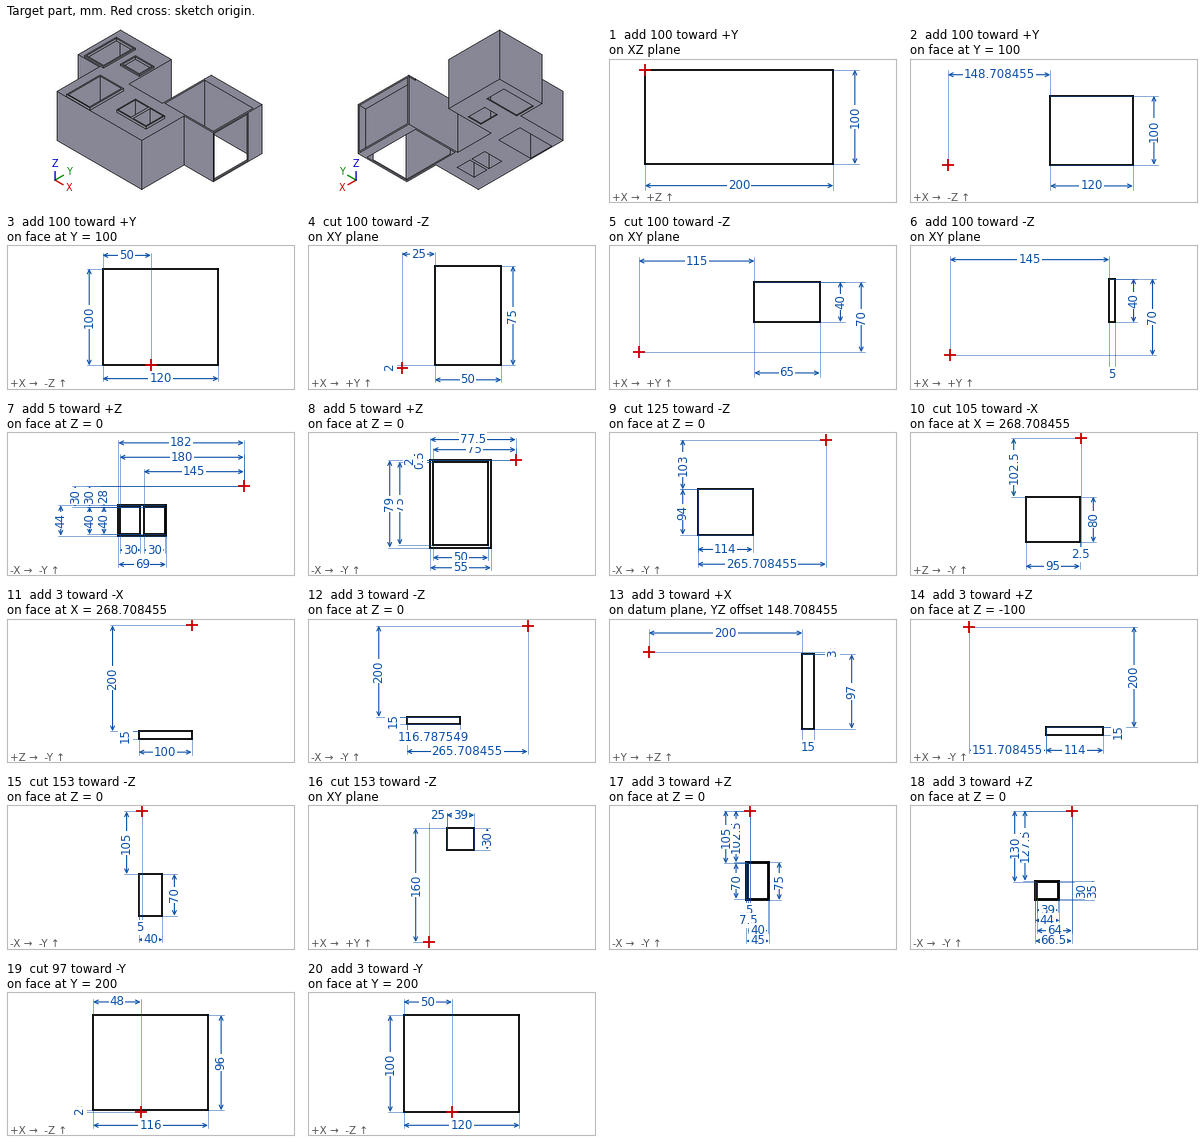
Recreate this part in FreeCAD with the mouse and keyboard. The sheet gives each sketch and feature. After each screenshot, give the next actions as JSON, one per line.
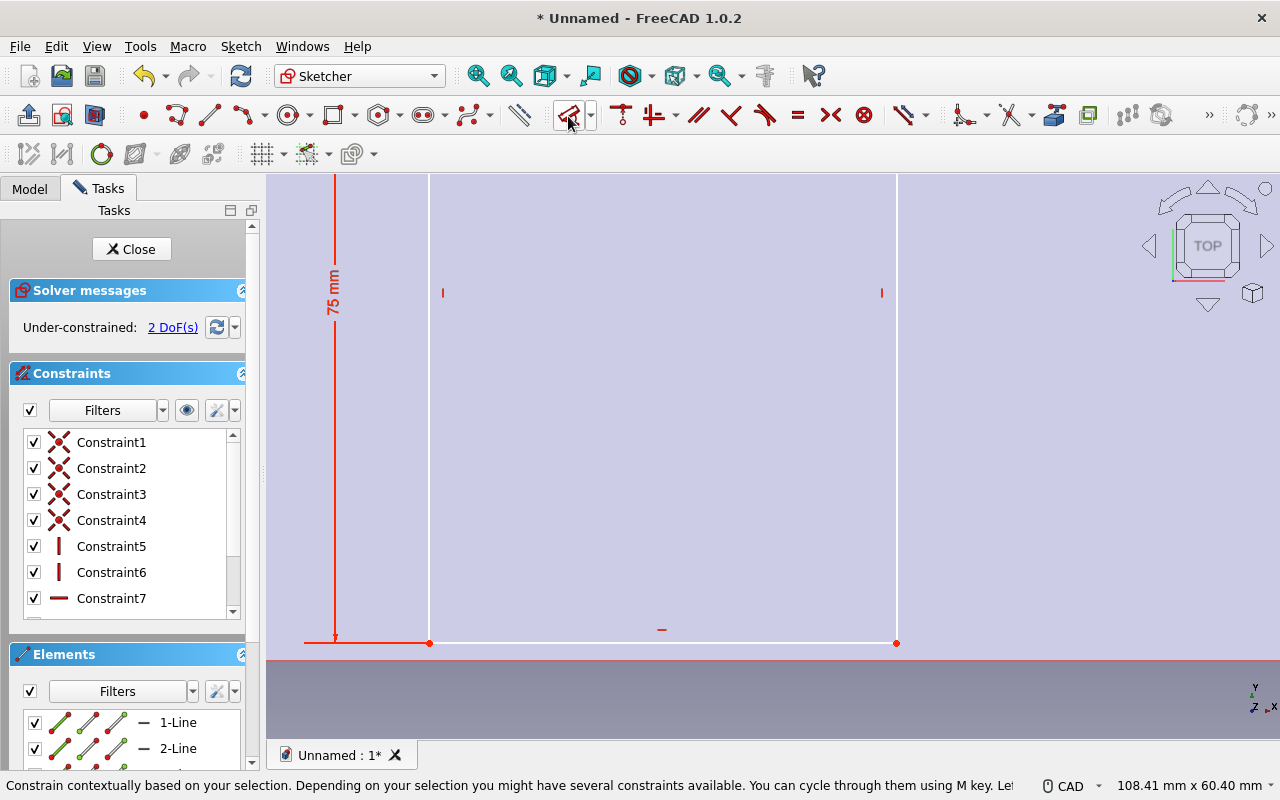
{"action": "scroll", "coordinate": [429, 643], "scroll_direction": "up", "scroll_amount": 4}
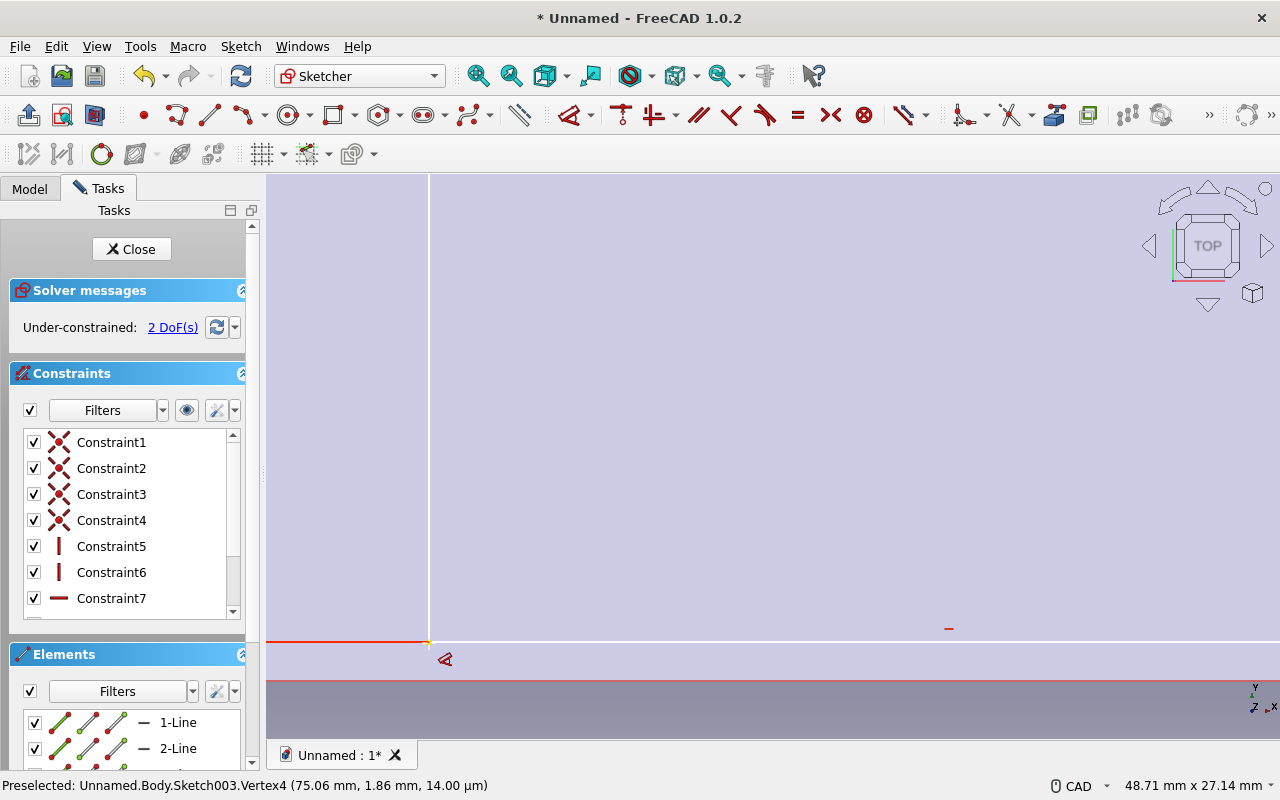
{"action": "left_click", "coordinate": [429, 642]}
{"action": "left_click", "coordinate": [463, 662]}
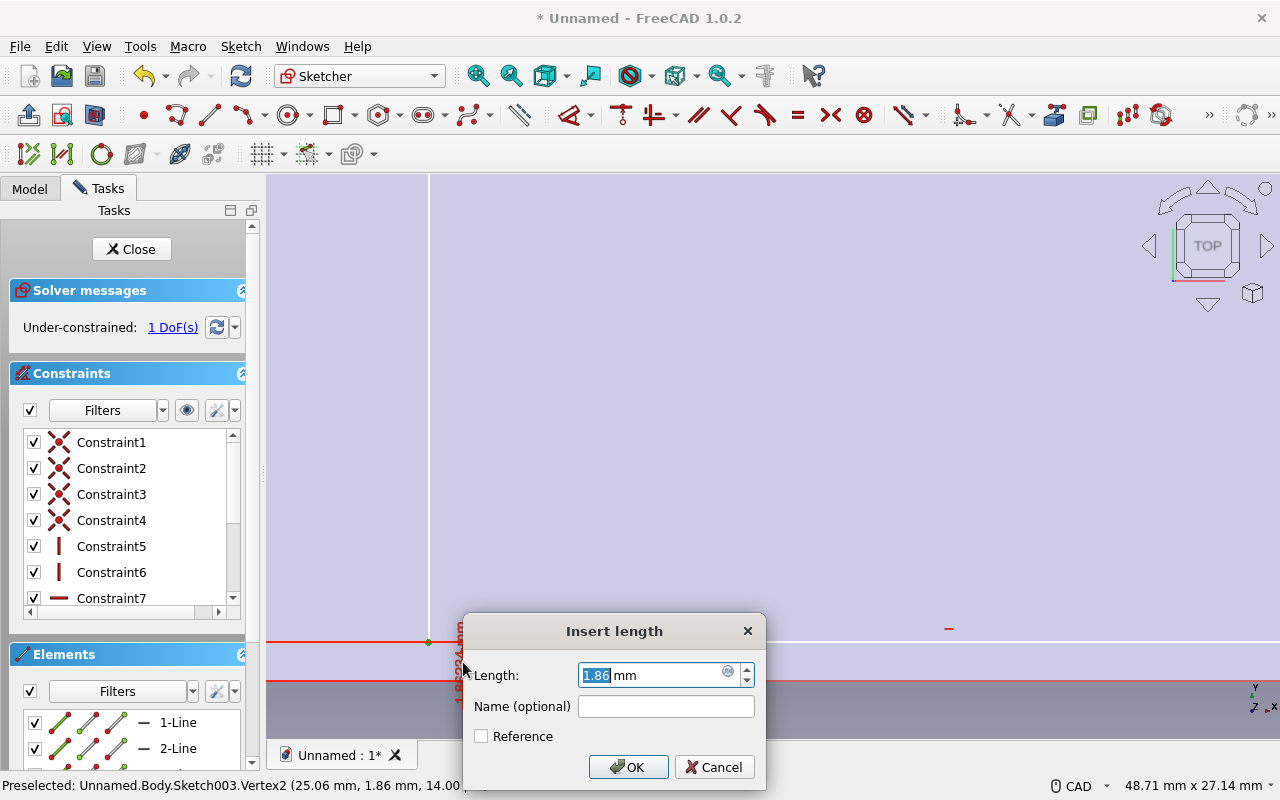
{"action": "type", "text": "2"}
{"action": "key", "text": "Return"}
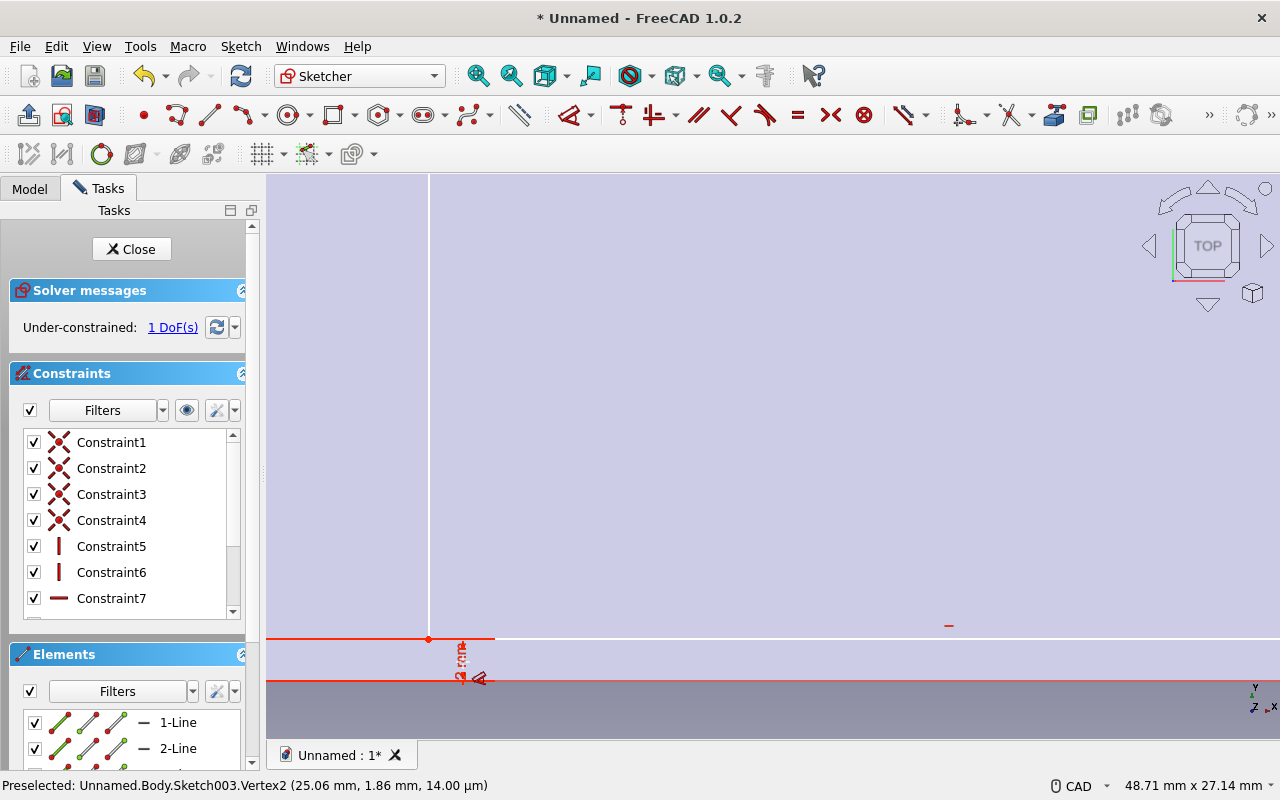
{"action": "scroll", "coordinate": [710, 645], "scroll_direction": "down", "scroll_amount": 7}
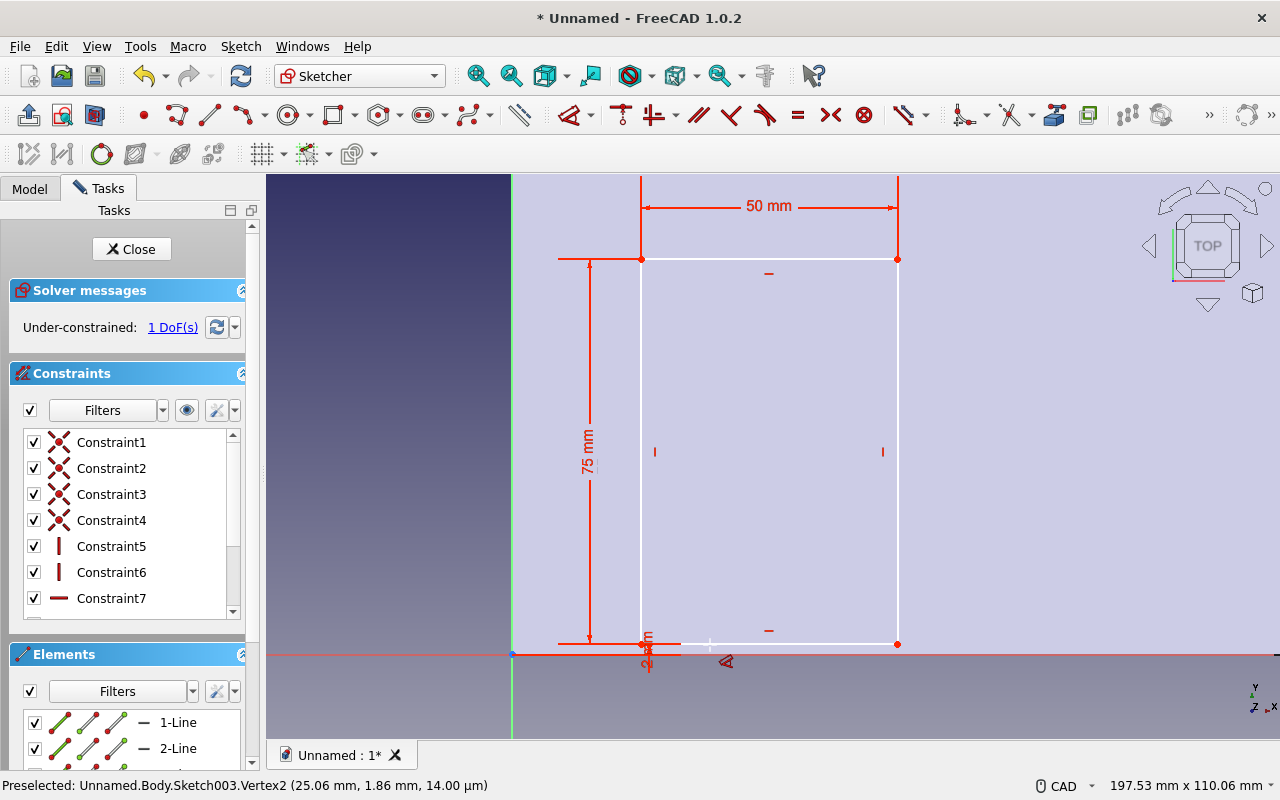
{"action": "left_click", "coordinate": [641, 259]}
{"action": "left_click", "coordinate": [577, 689]}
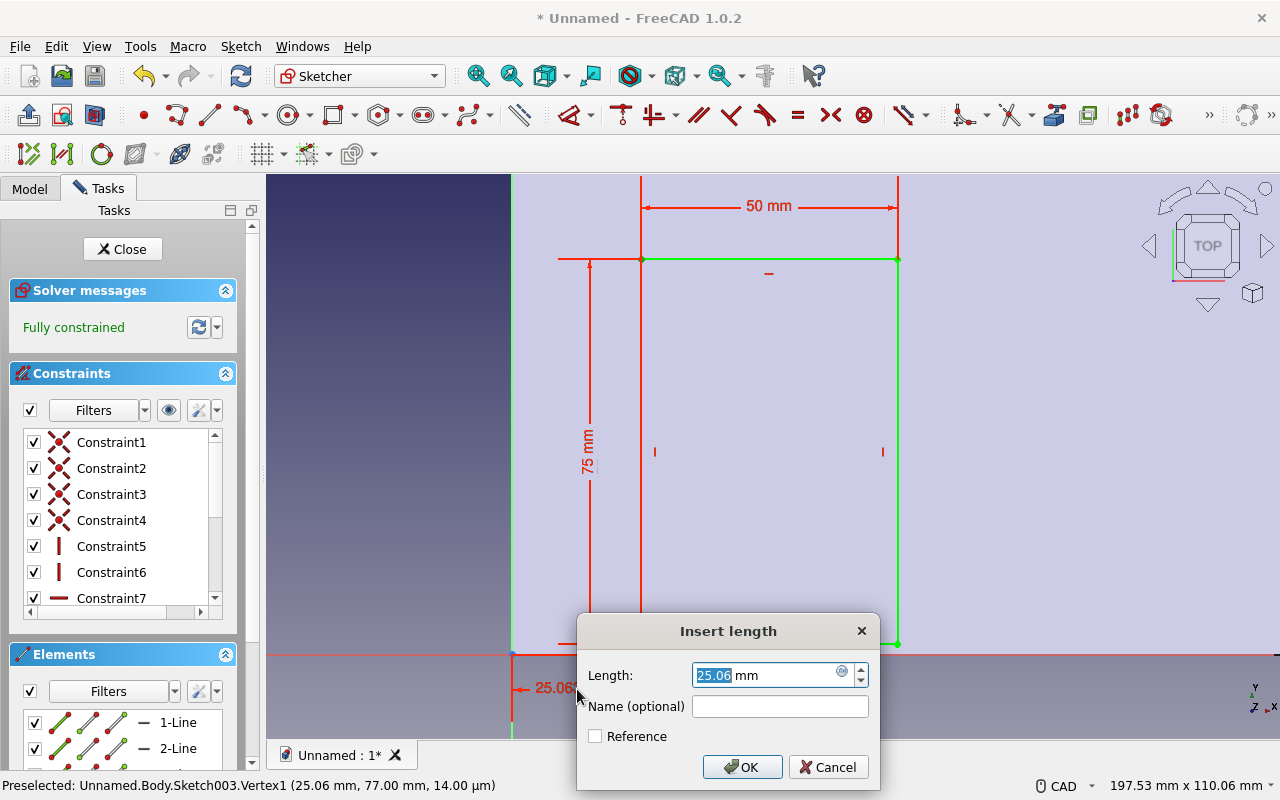
{"action": "type", "text": "25"}
{"action": "key", "text": "Return"}
{"action": "key", "text": "Escape"}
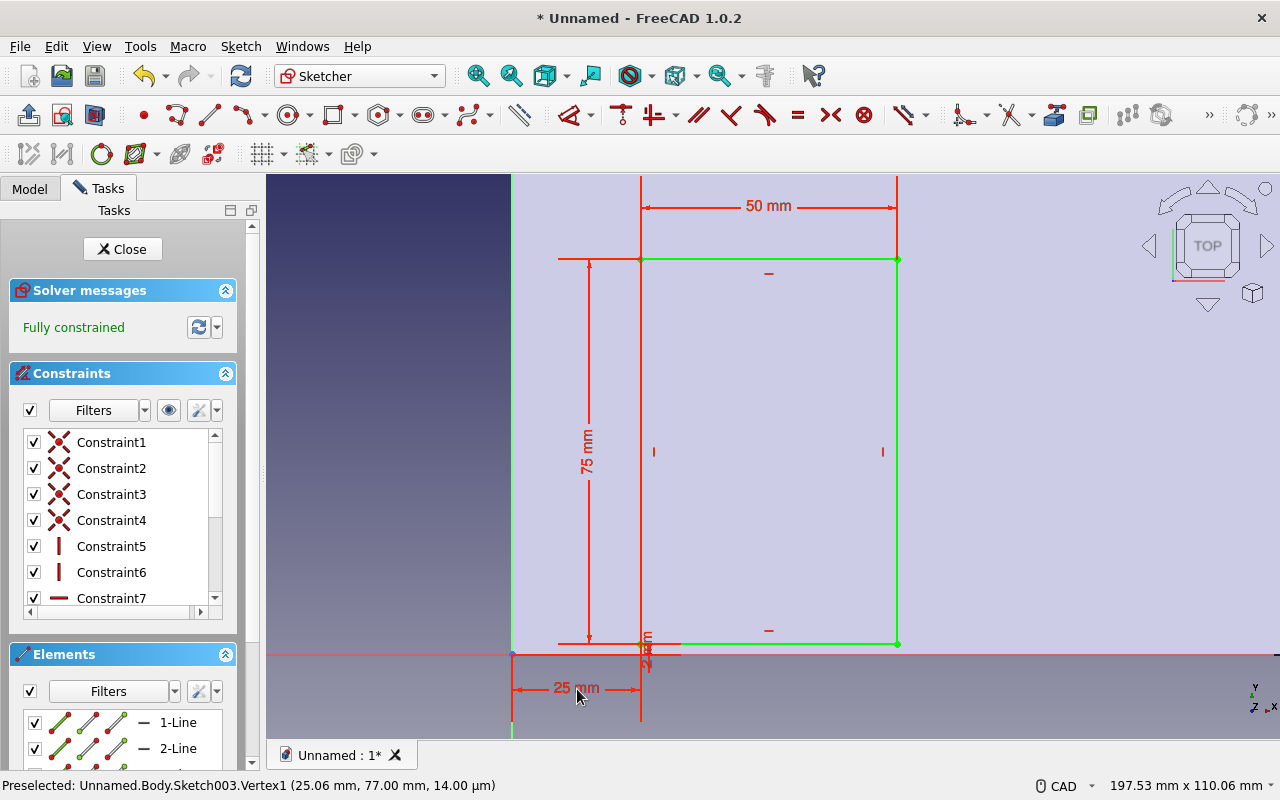
{"action": "left_click", "coordinate": [123, 249]}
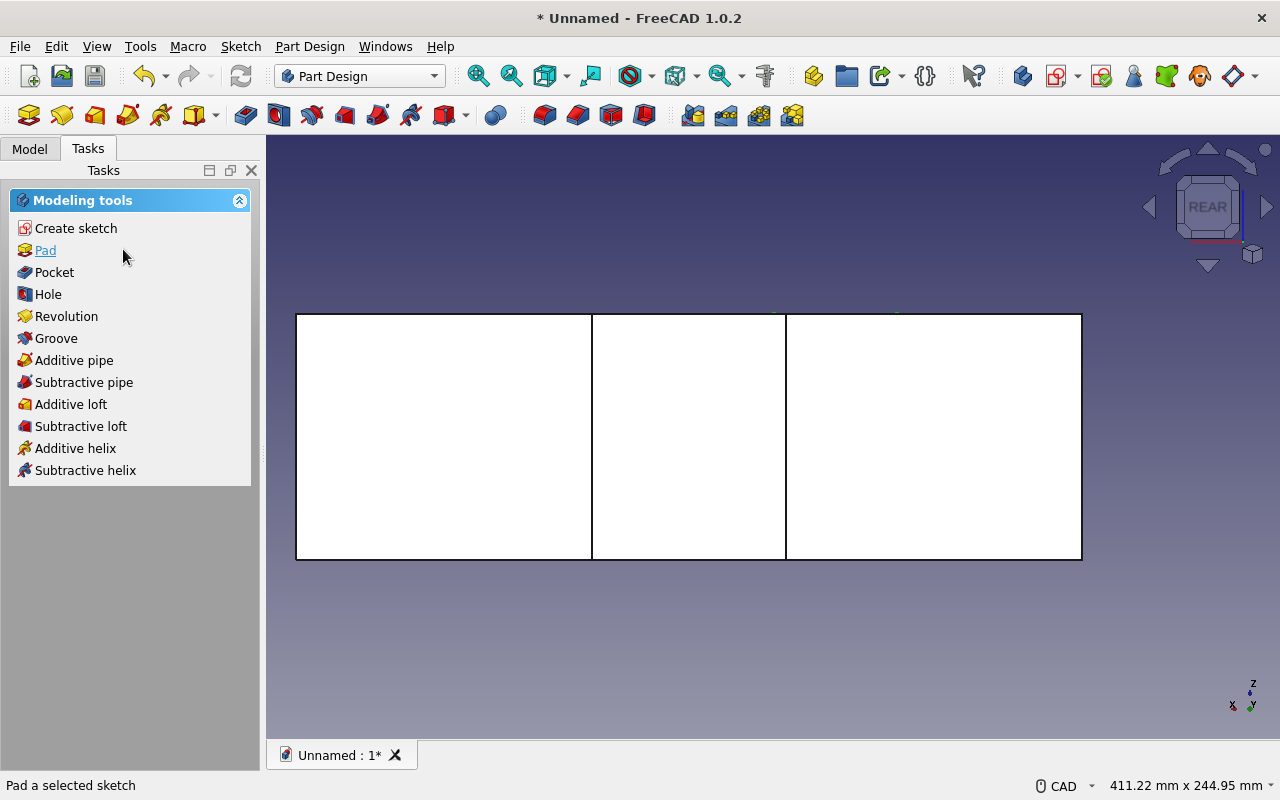
{"action": "left_click", "coordinate": [246, 116]}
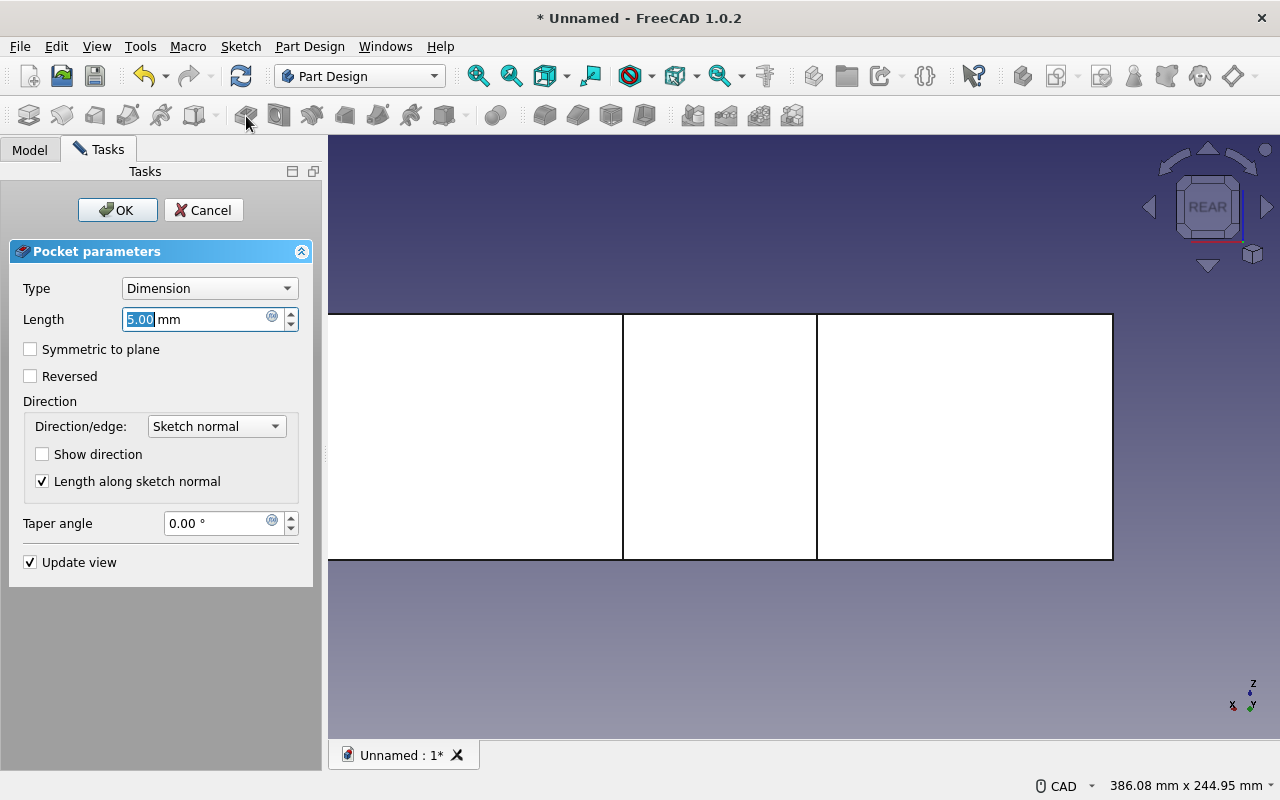
{"action": "type", "text": "100"}
{"action": "key", "text": "Tab"}